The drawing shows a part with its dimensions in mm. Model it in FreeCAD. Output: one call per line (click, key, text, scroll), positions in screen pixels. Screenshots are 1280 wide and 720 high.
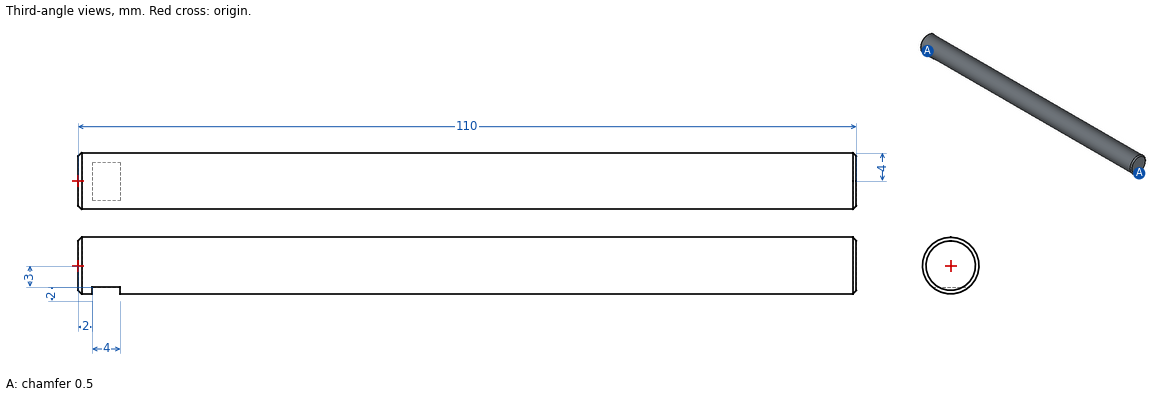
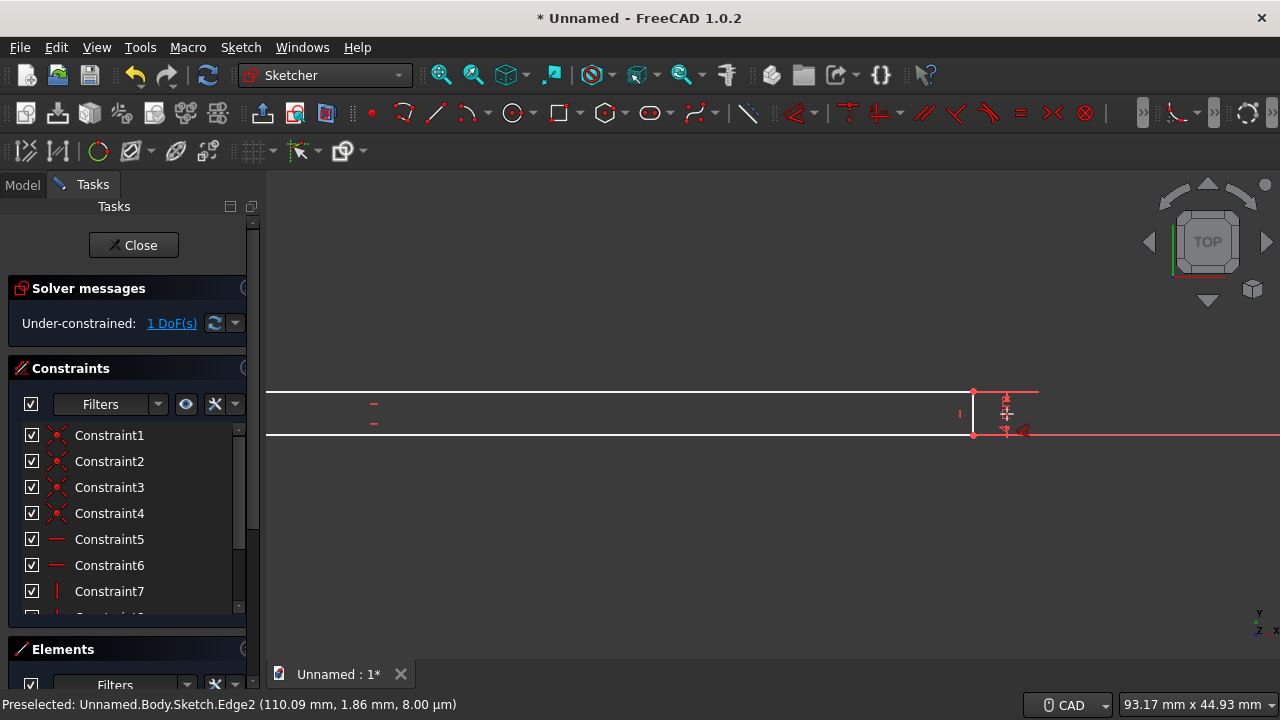
click(614, 435)
click(634, 469)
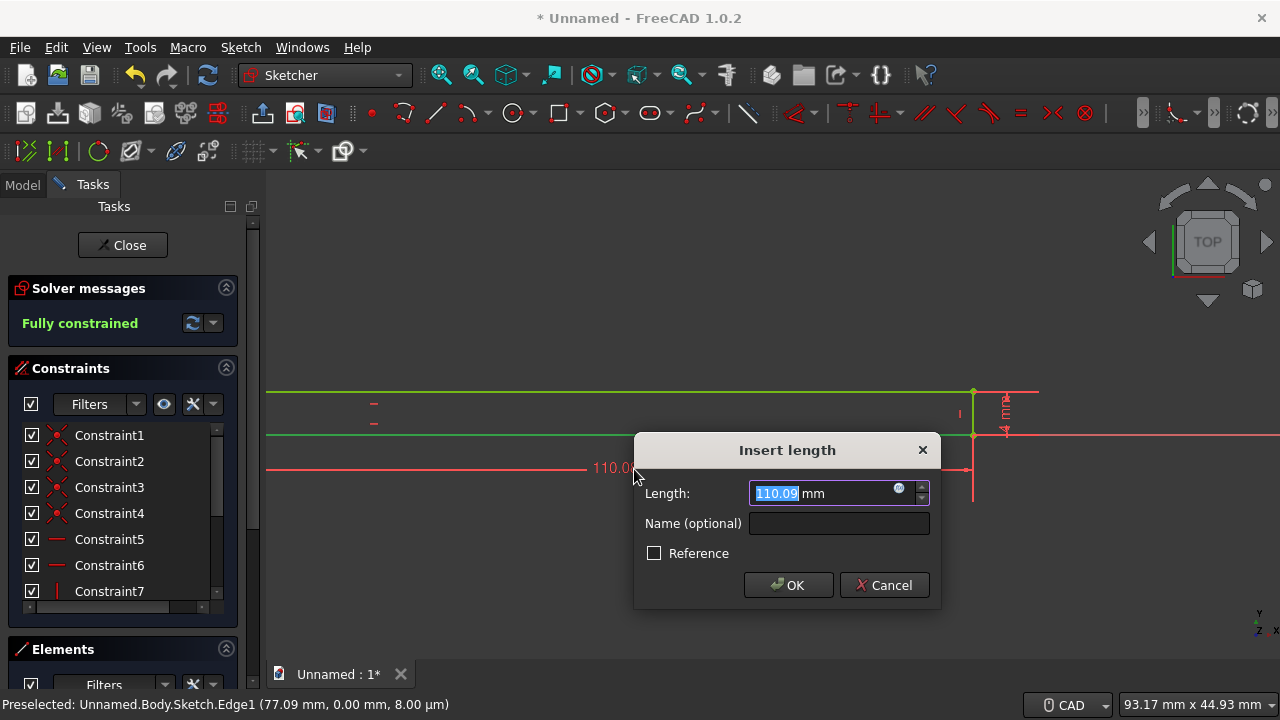
text(110)
key(Return)
key(Escape)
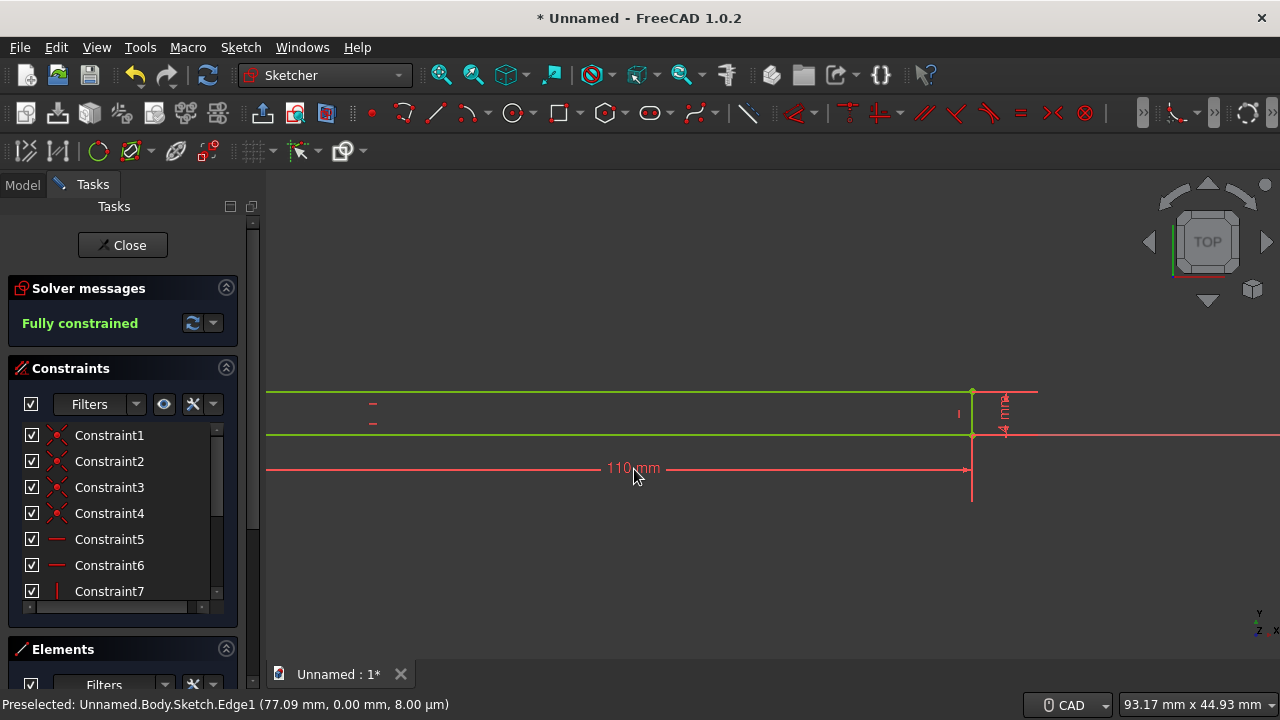
click(123, 245)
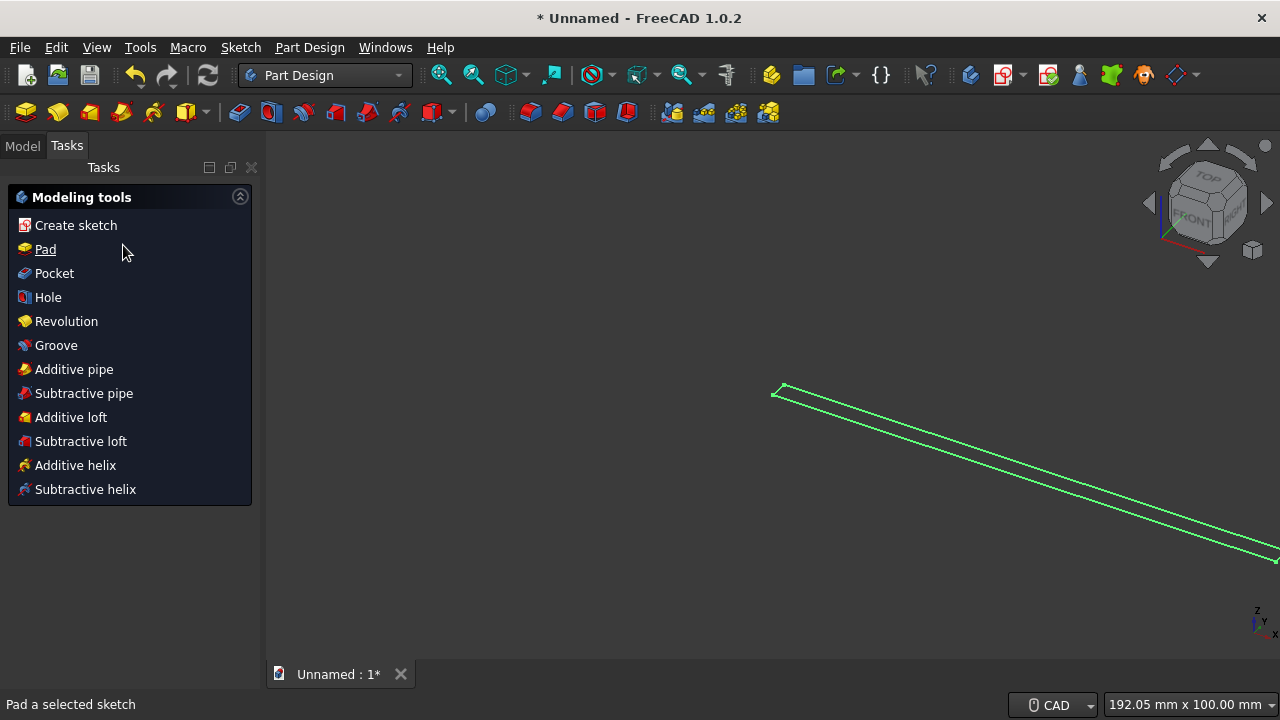
click(58, 112)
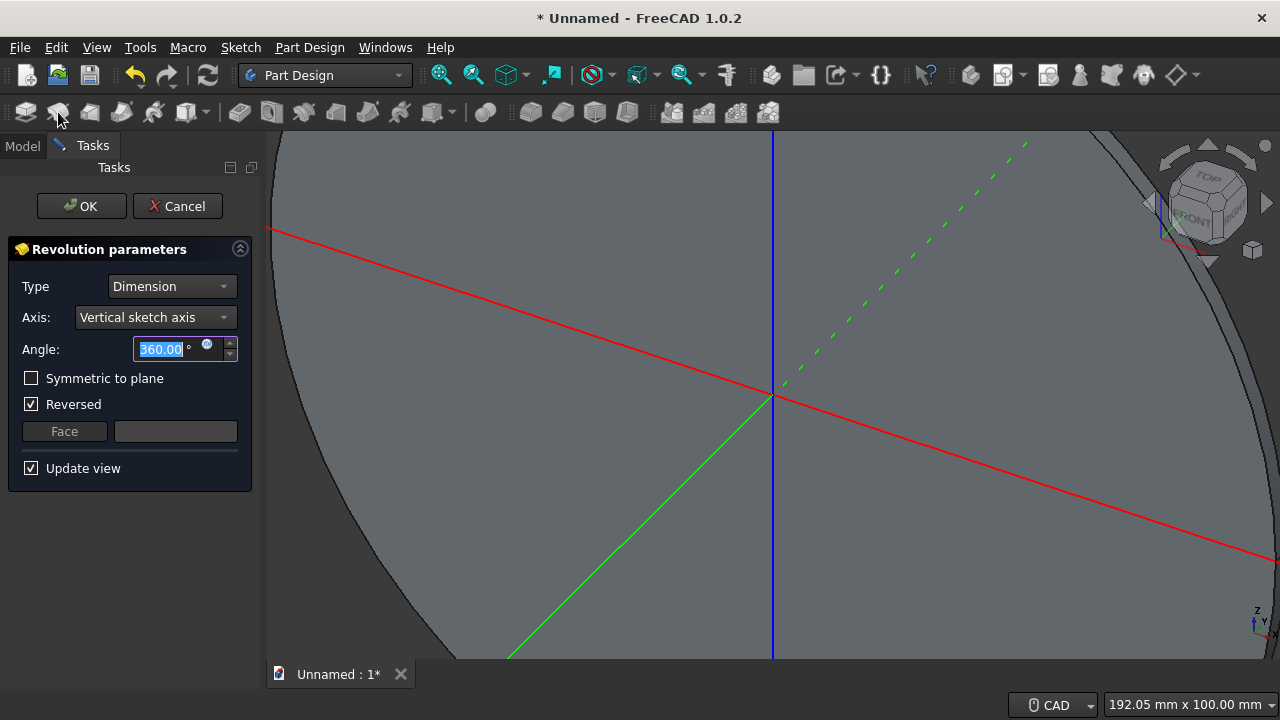
click(156, 318)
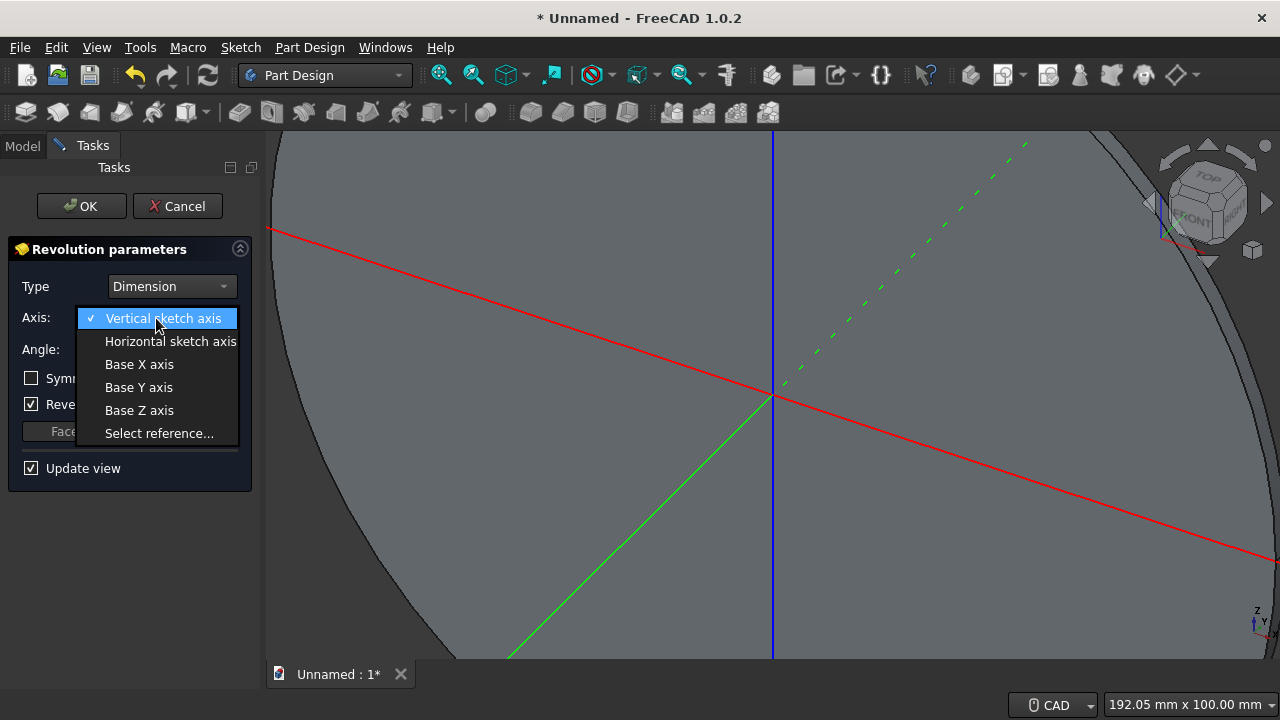
click(156, 342)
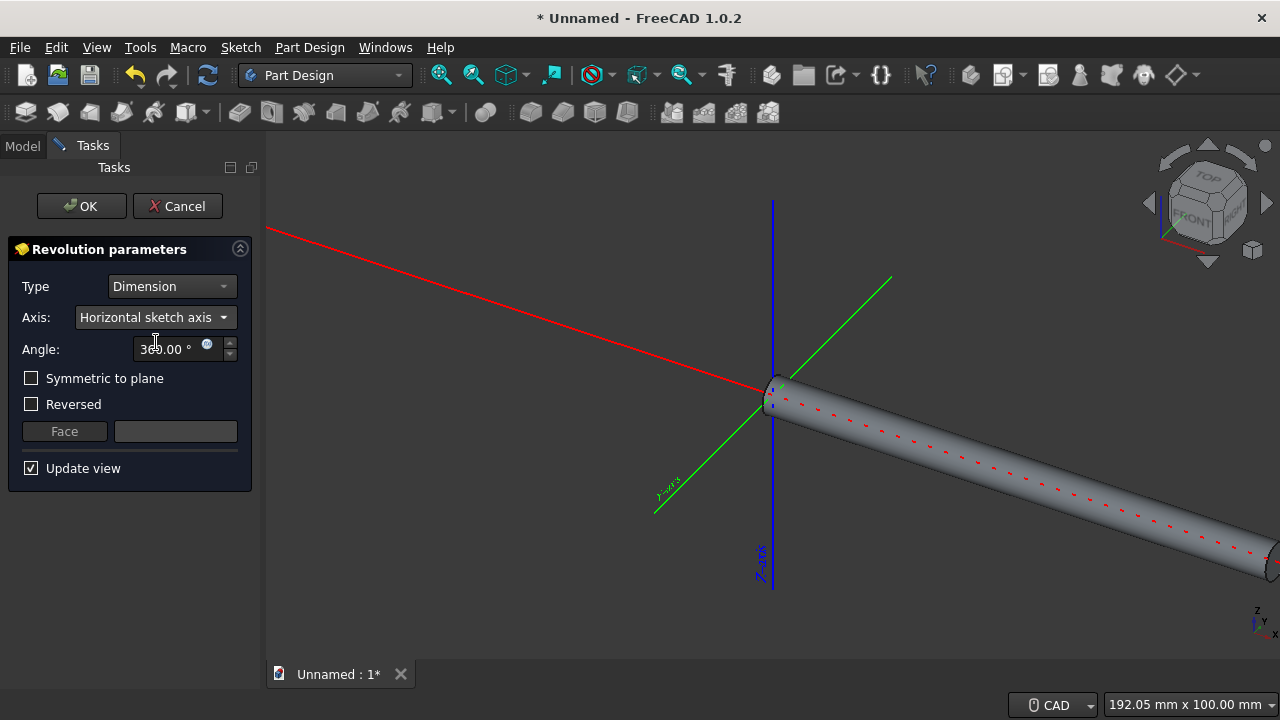
click(82, 206)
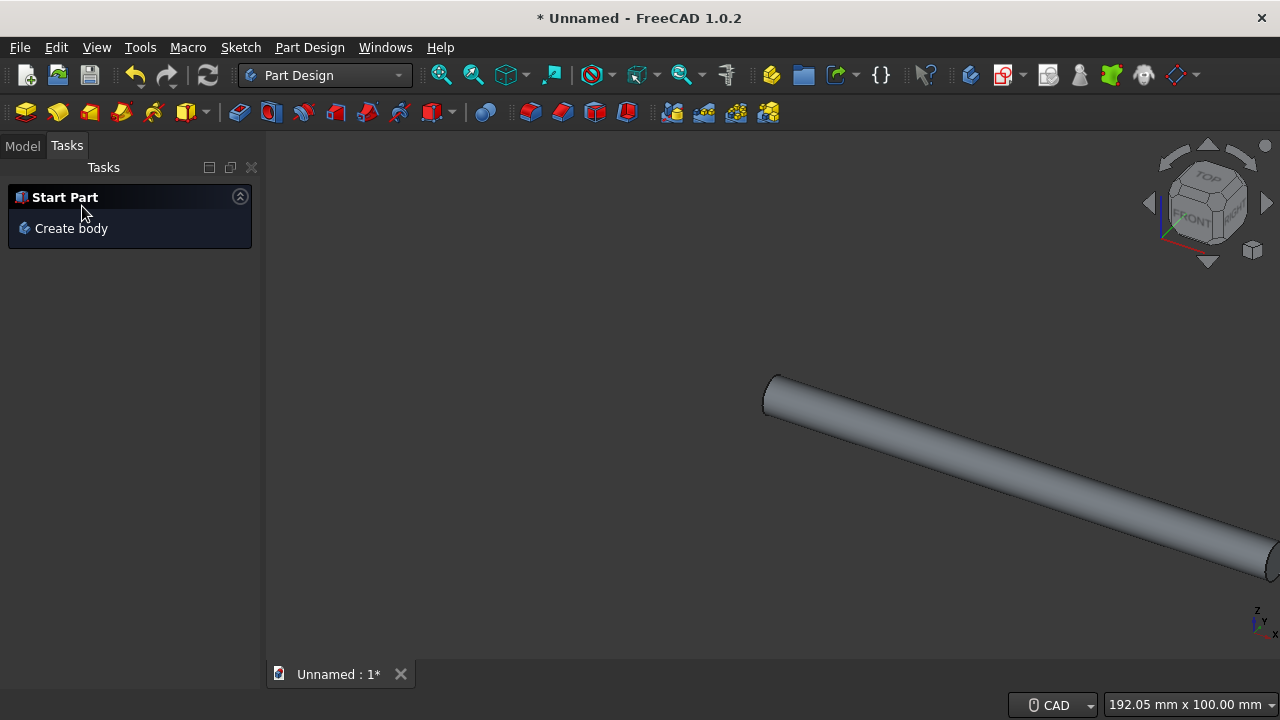
click(442, 76)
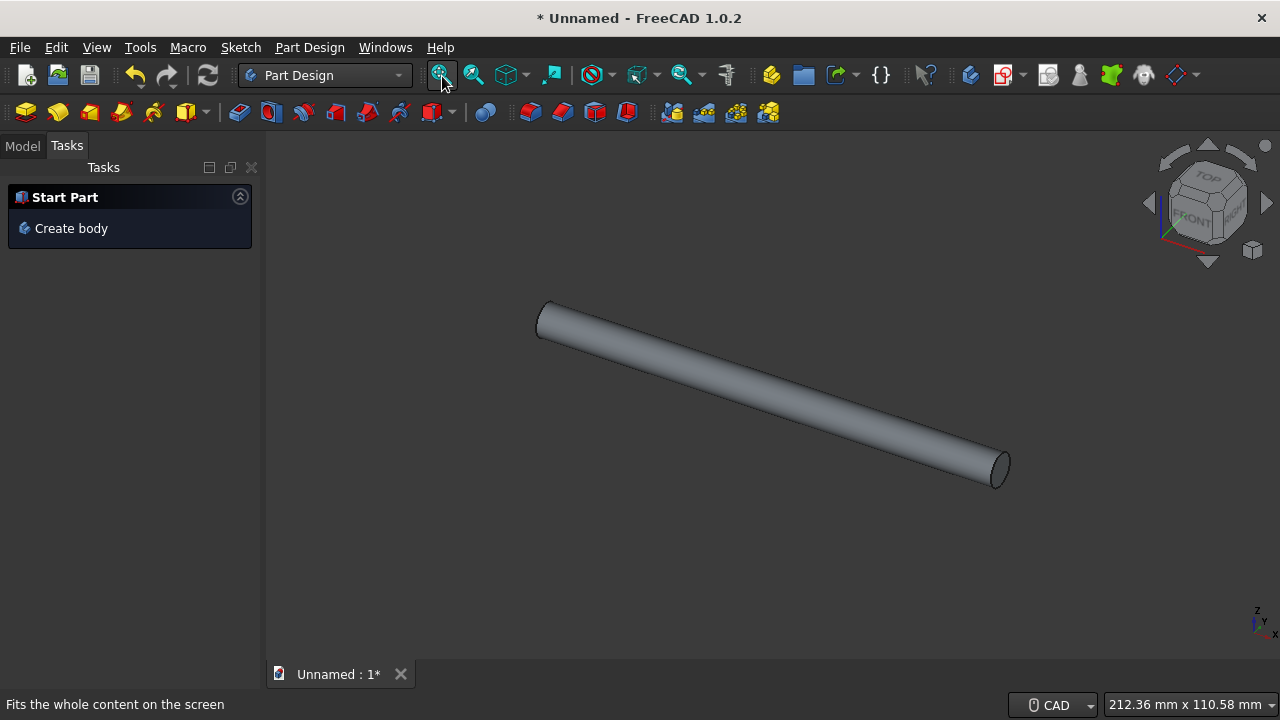
click(1004, 76)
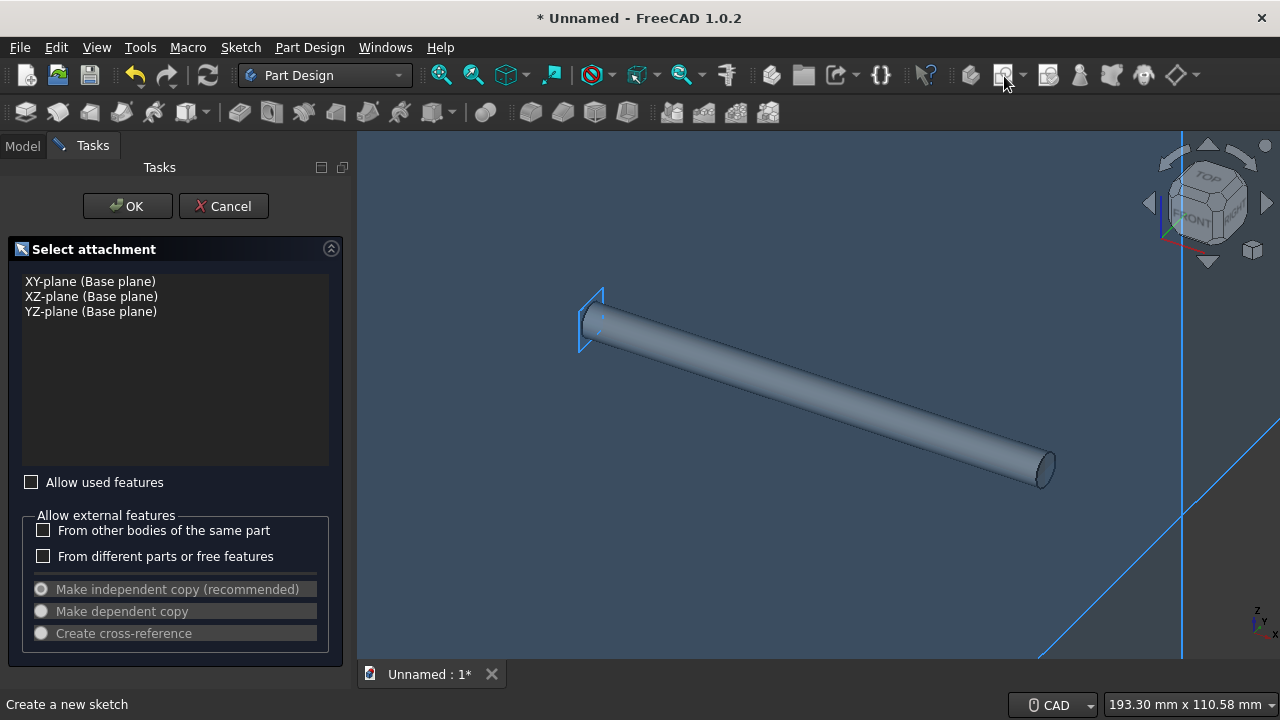
click(82, 296)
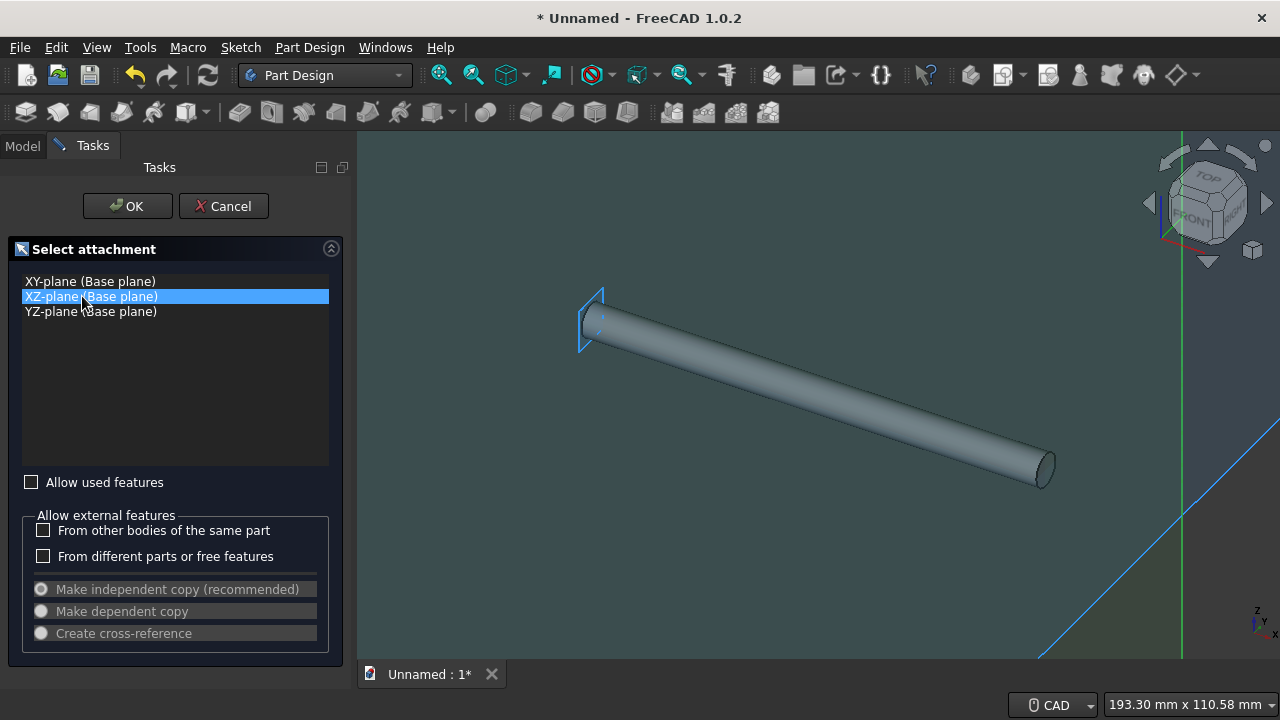
click(128, 206)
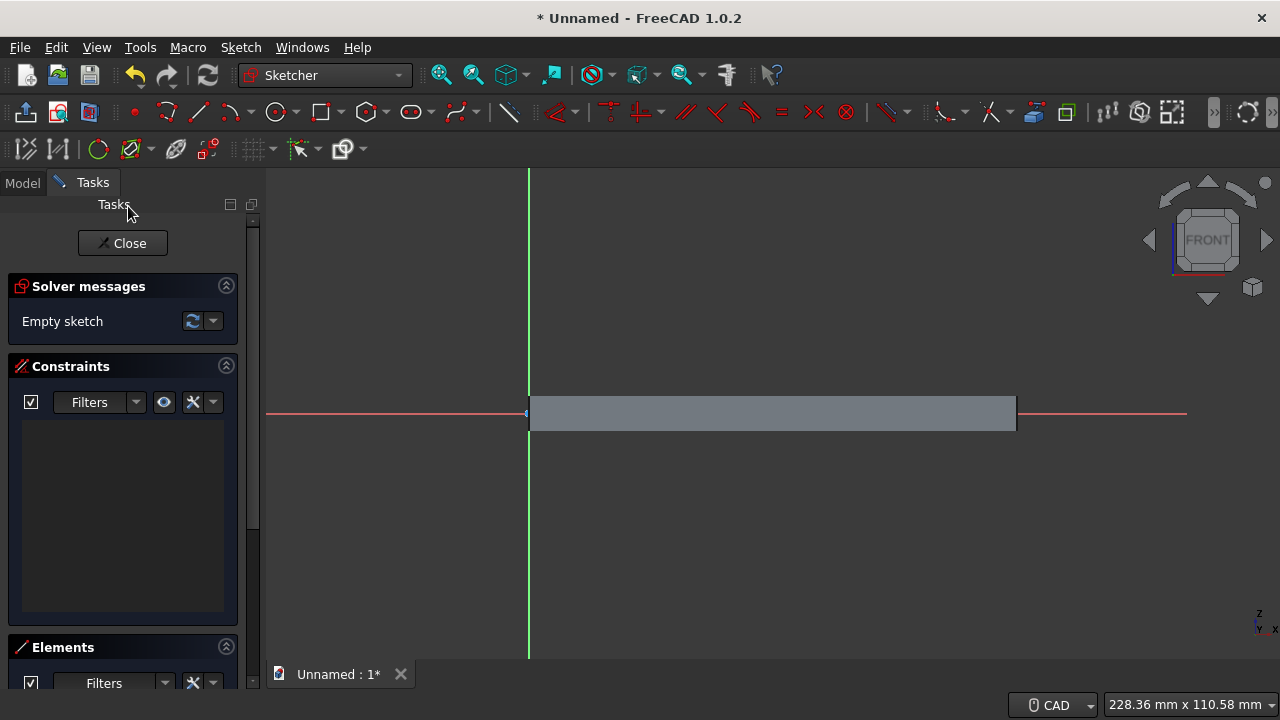
click(90, 112)